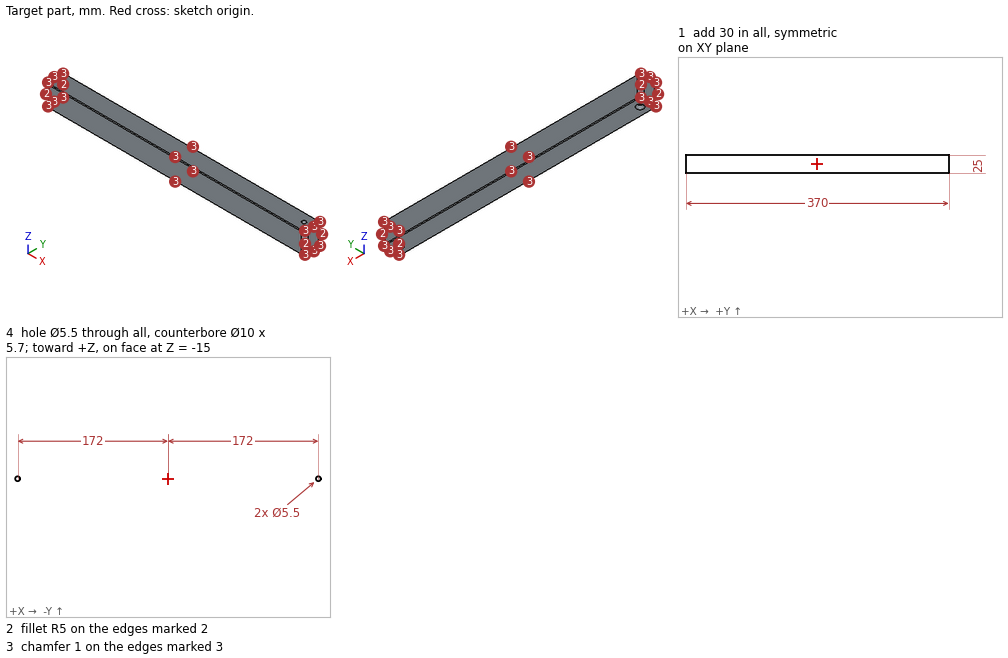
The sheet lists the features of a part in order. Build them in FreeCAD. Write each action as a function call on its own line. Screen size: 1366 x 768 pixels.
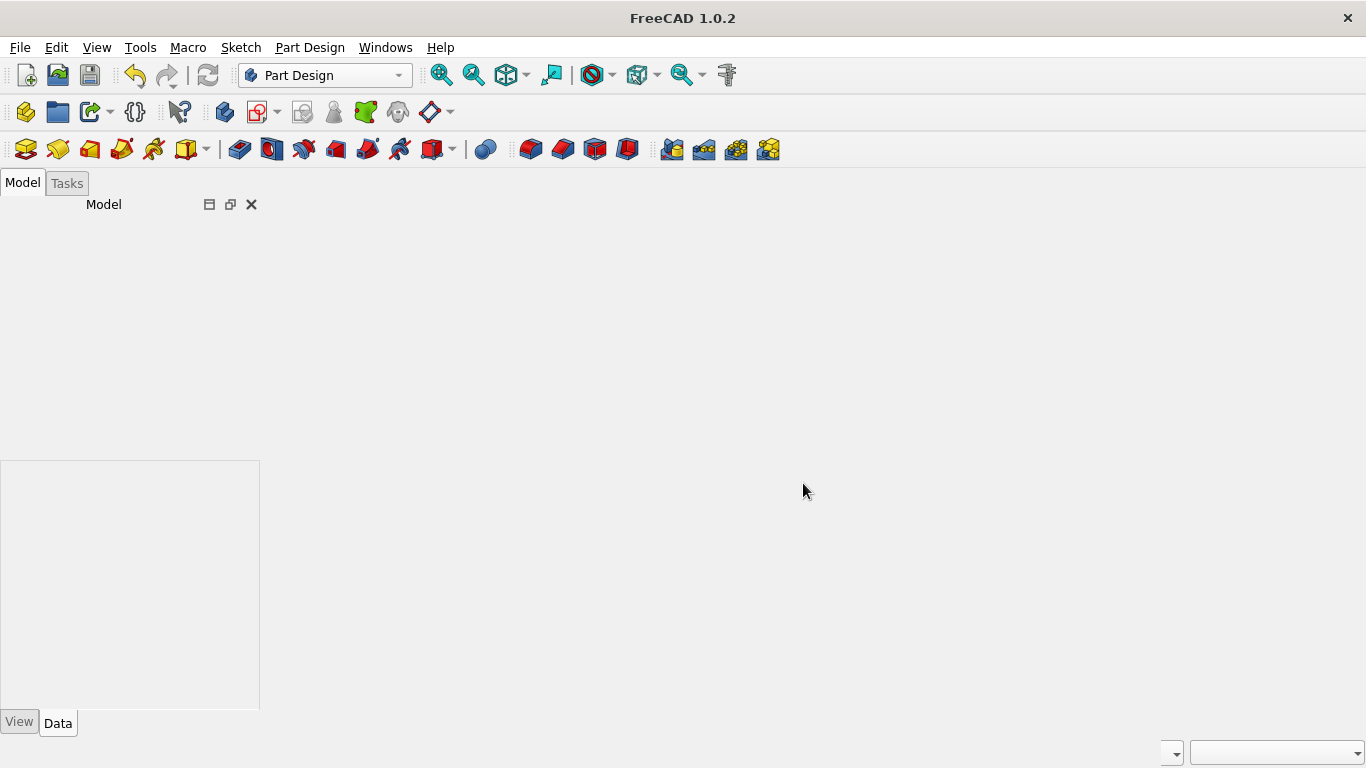
click(26, 76)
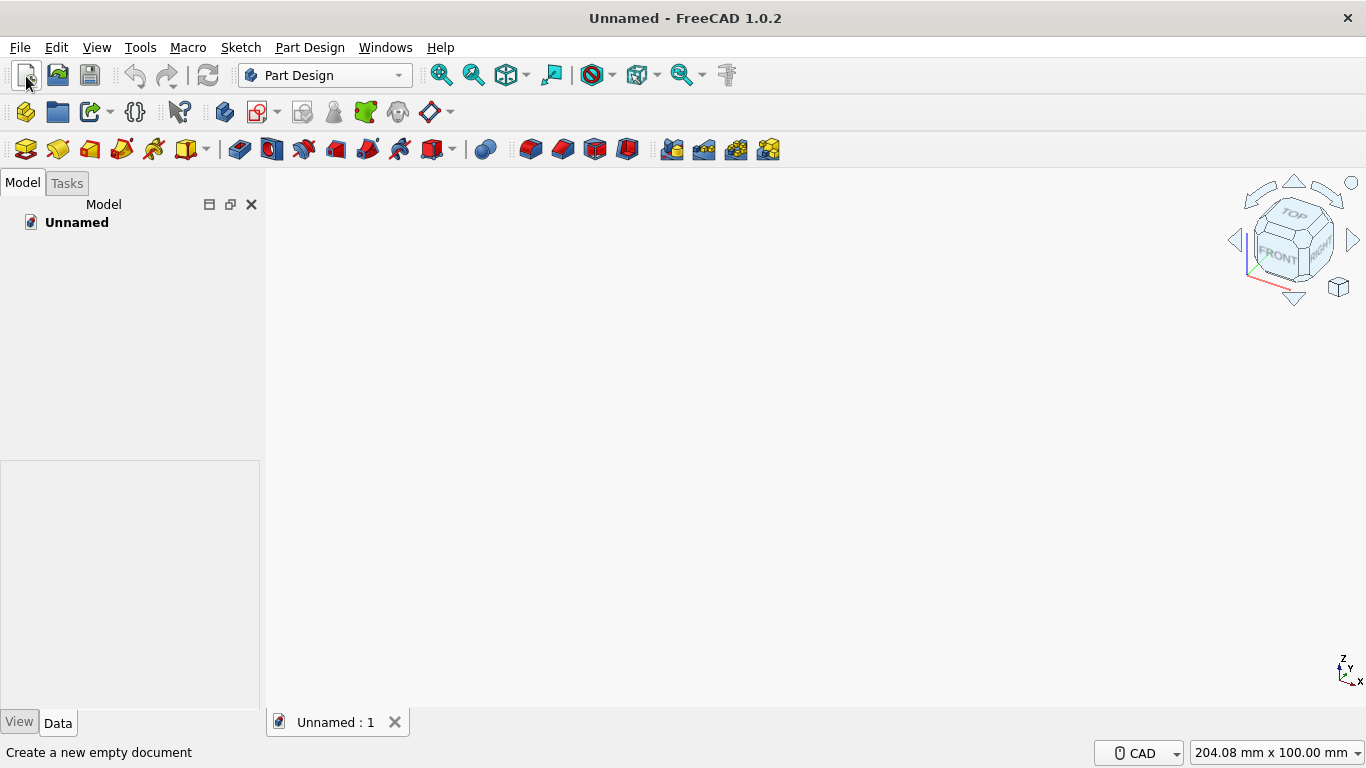
click(258, 112)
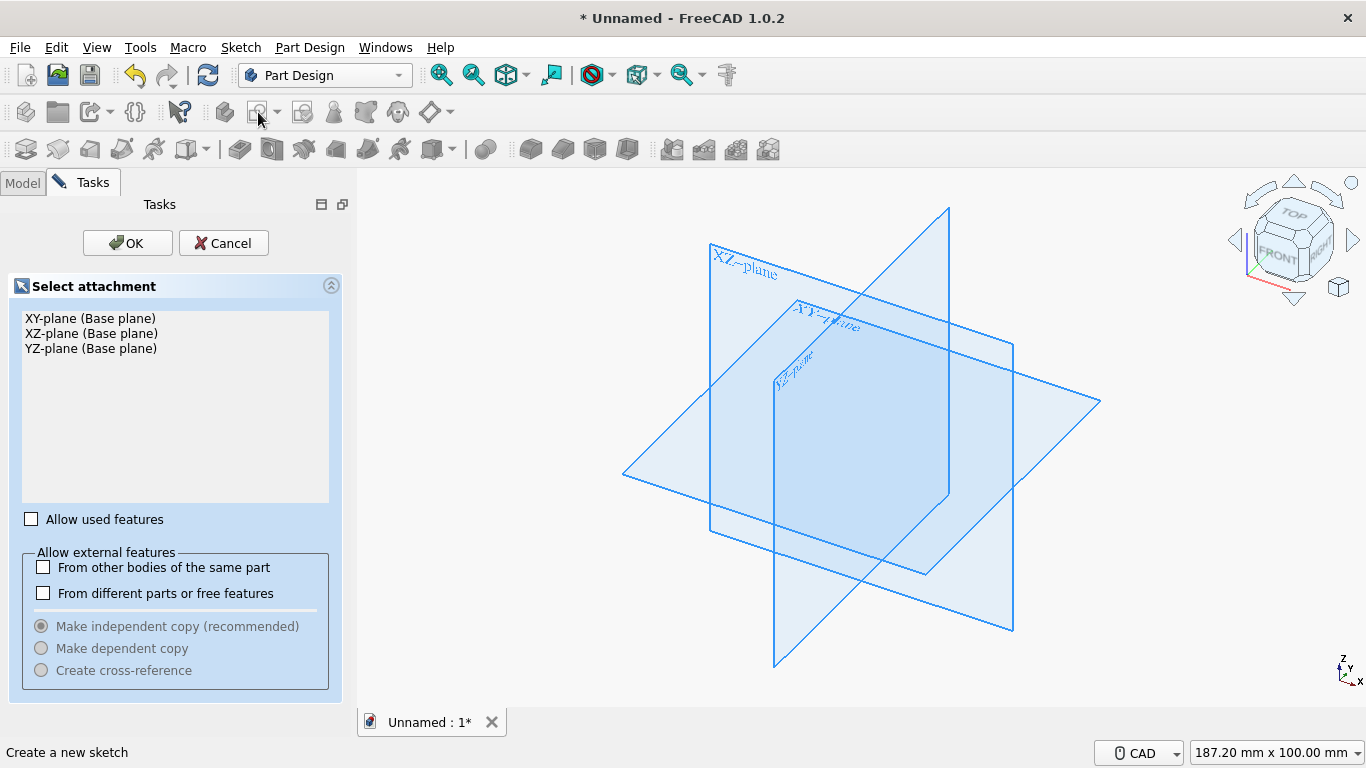
click(82, 318)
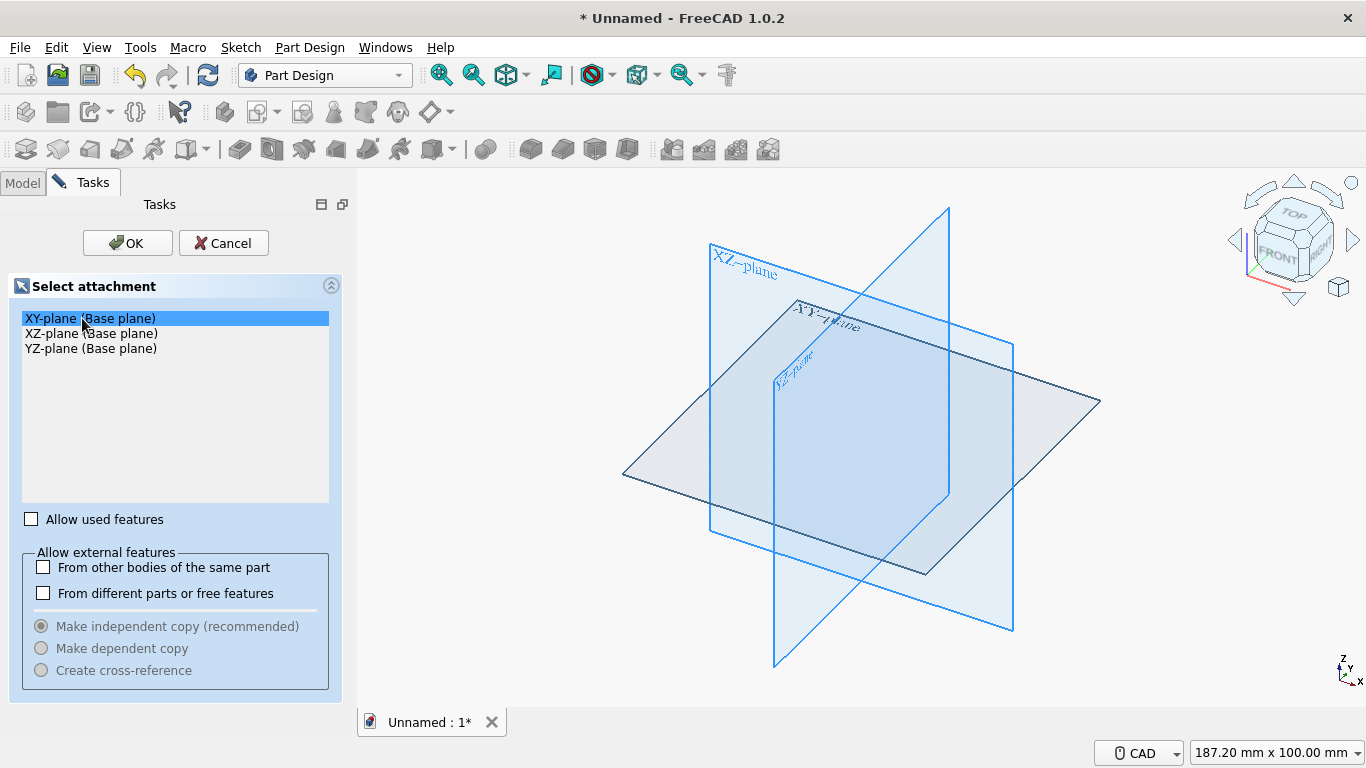
click(128, 243)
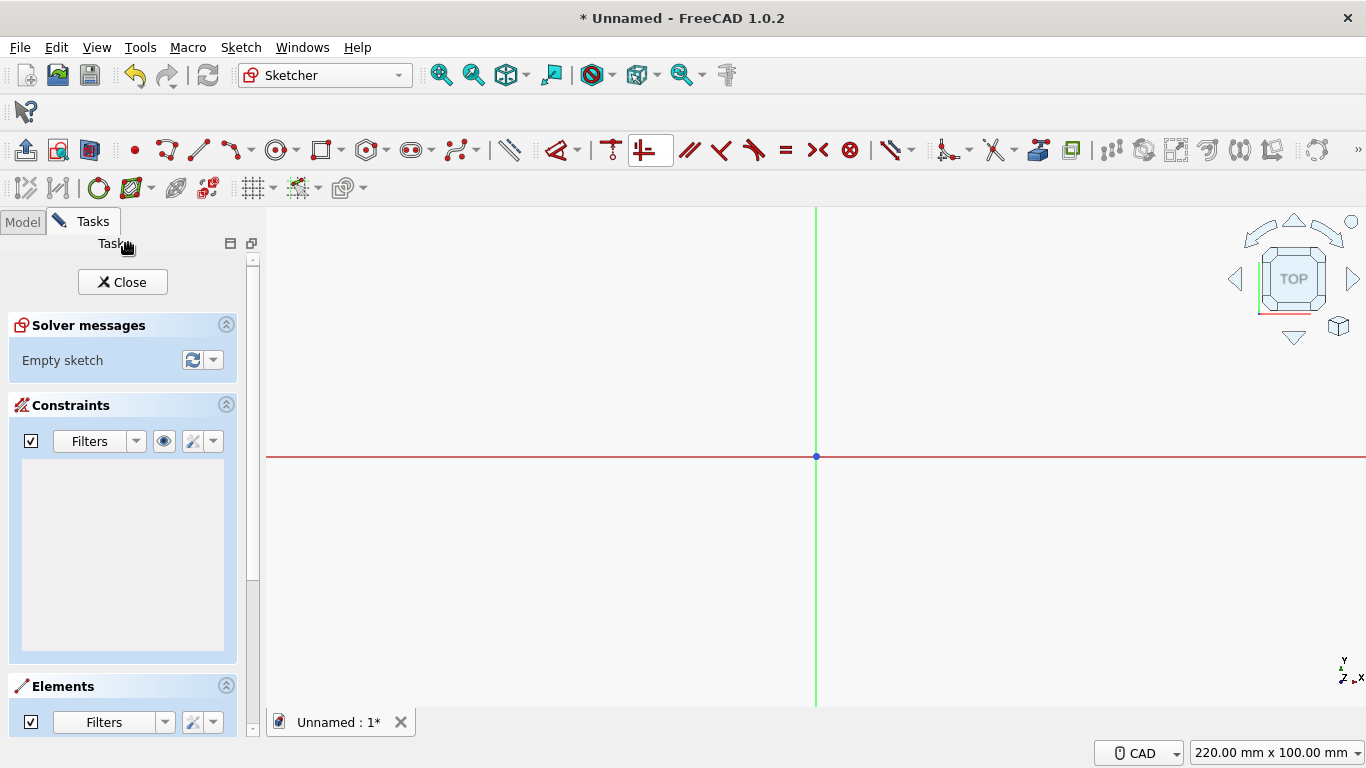
scroll(708, 457, down, 5)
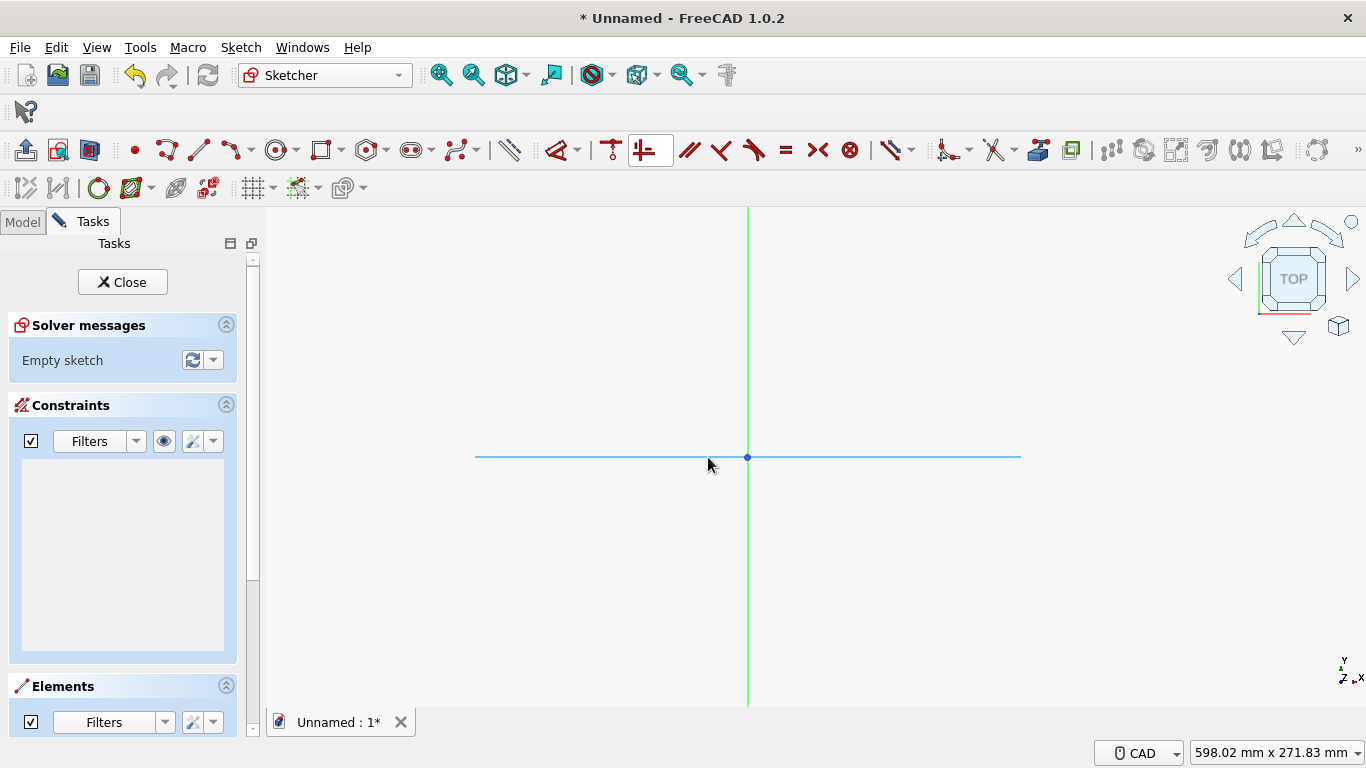
key(g)
key(v)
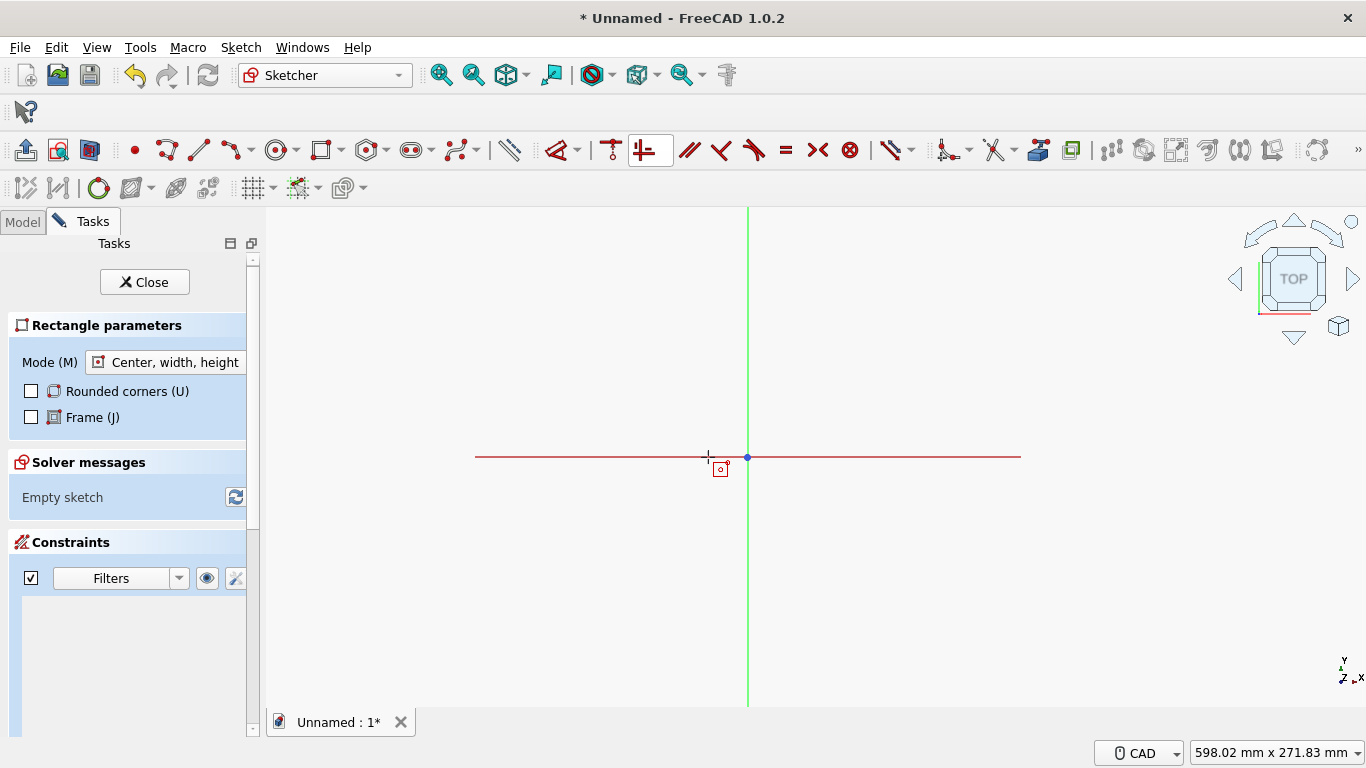
click(748, 457)
click(1088, 434)
key(Escape)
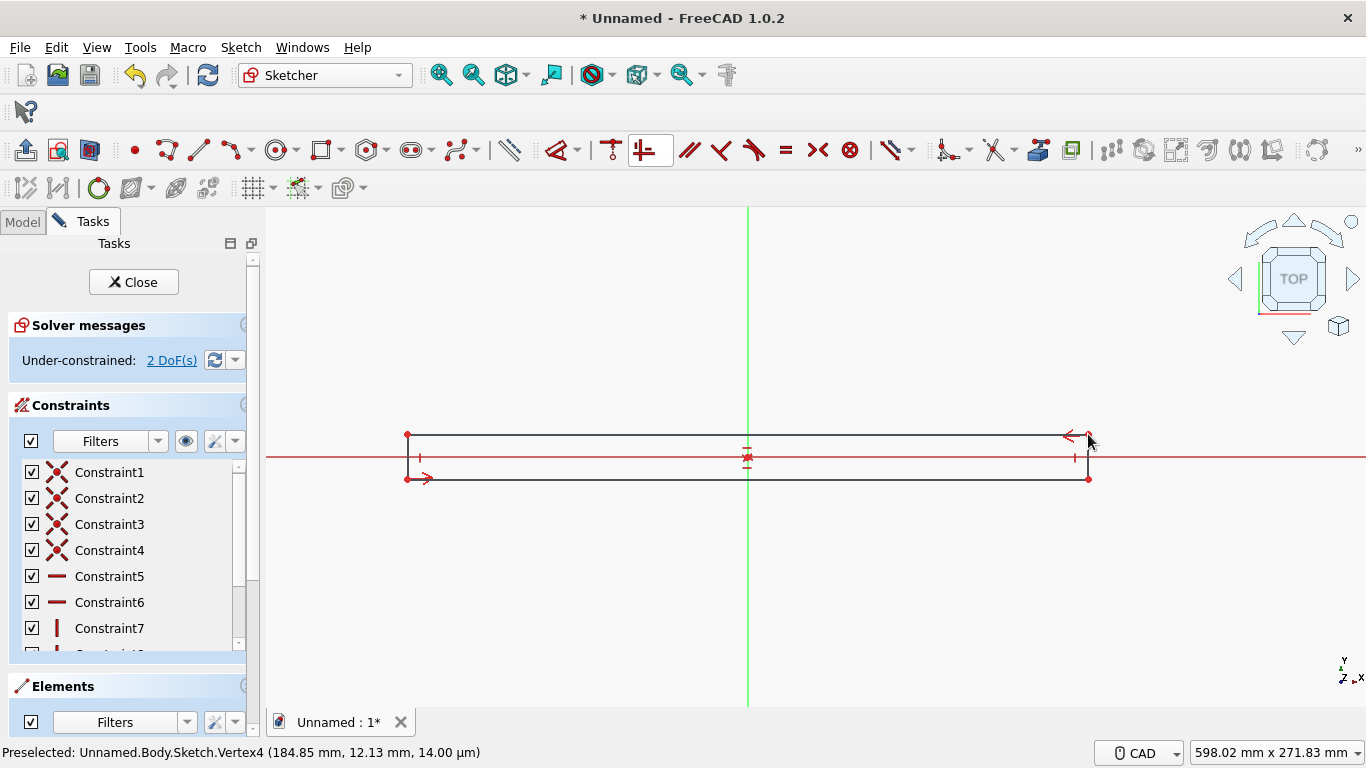
click(556, 150)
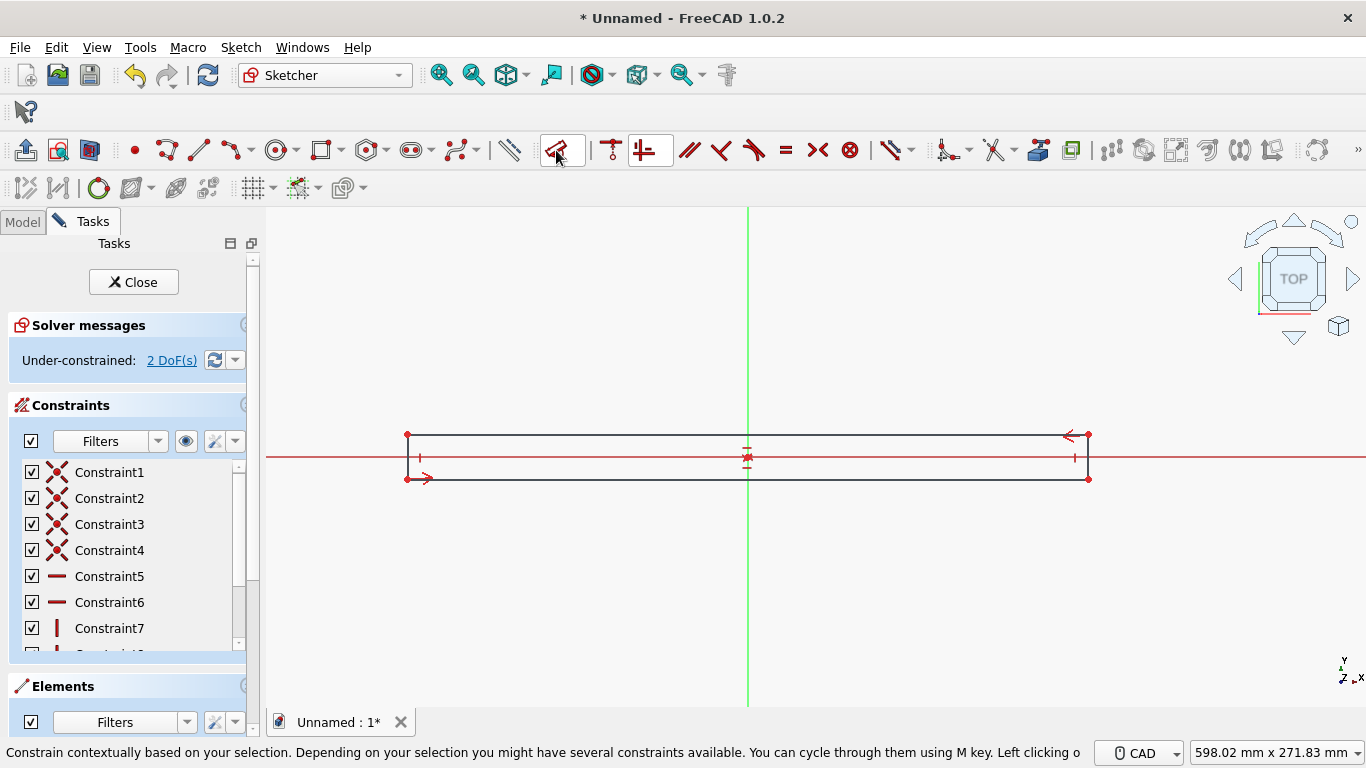
click(1088, 457)
click(1122, 442)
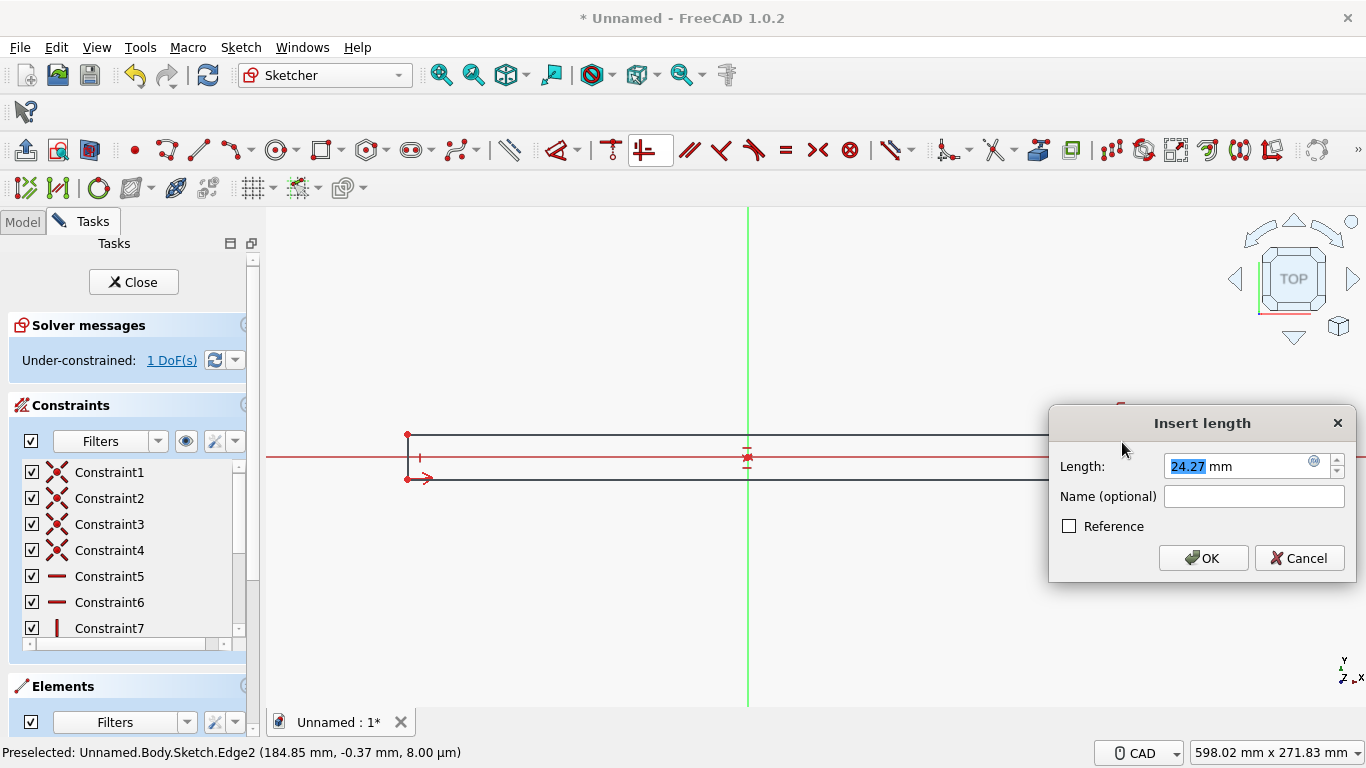
text(25)
key(Return)